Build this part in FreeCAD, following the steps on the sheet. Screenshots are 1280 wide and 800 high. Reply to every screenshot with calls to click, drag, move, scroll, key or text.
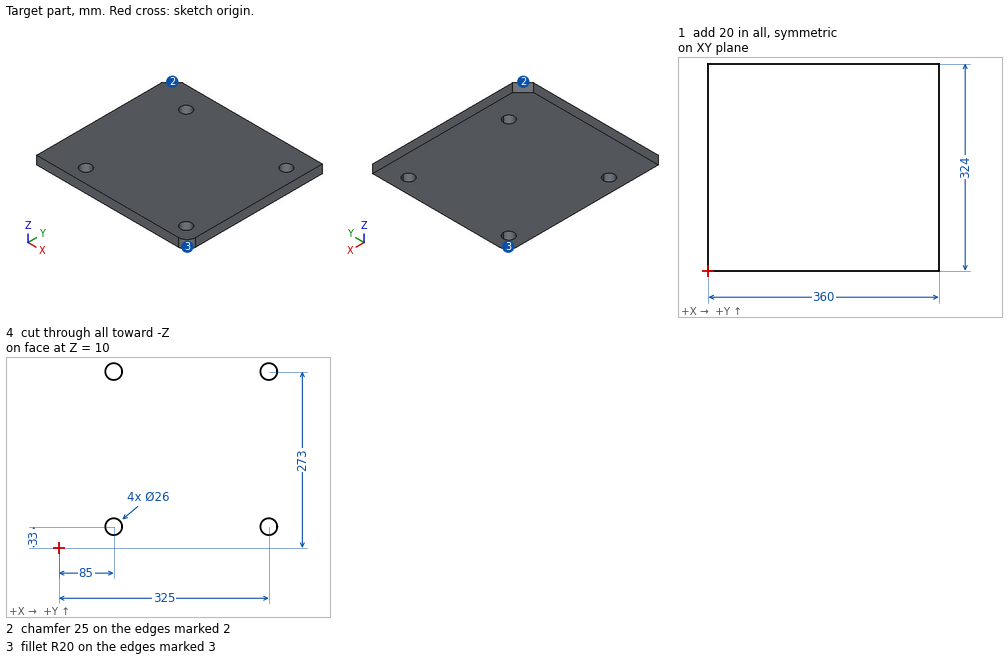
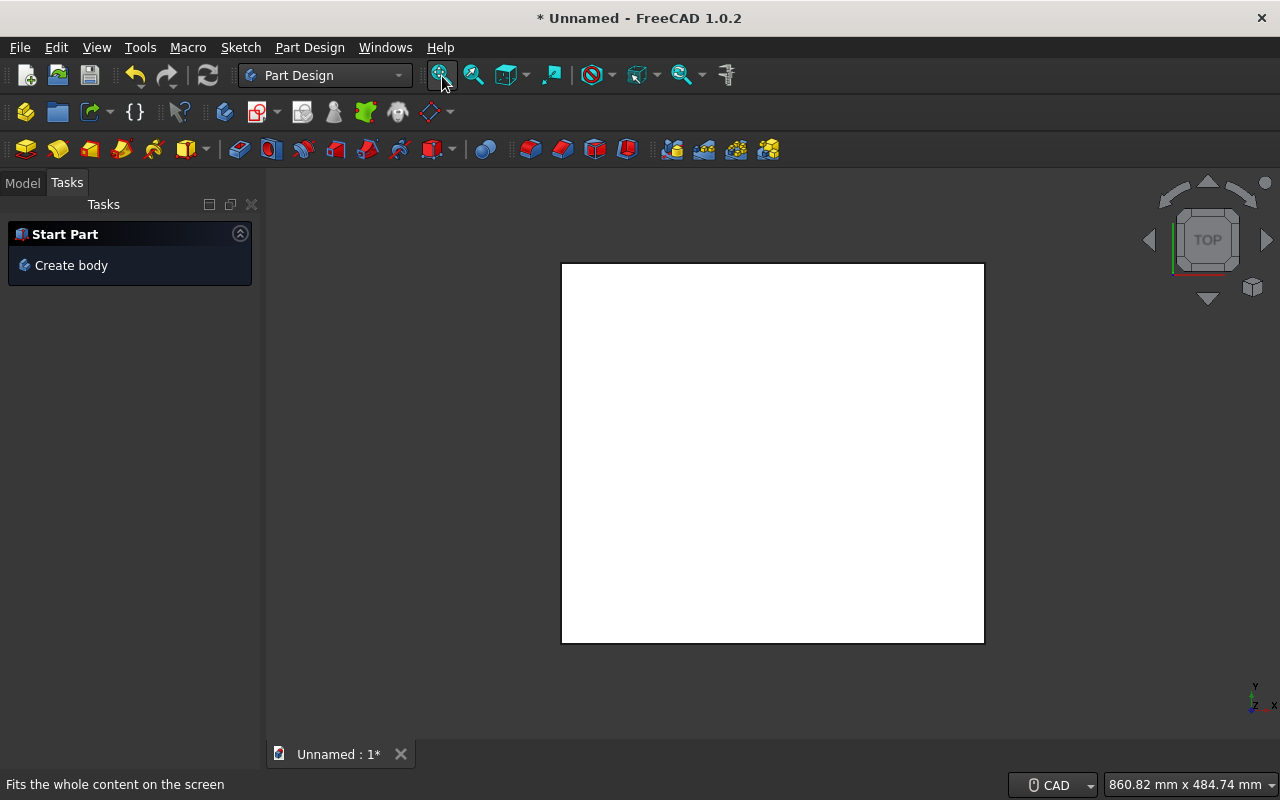
key(1)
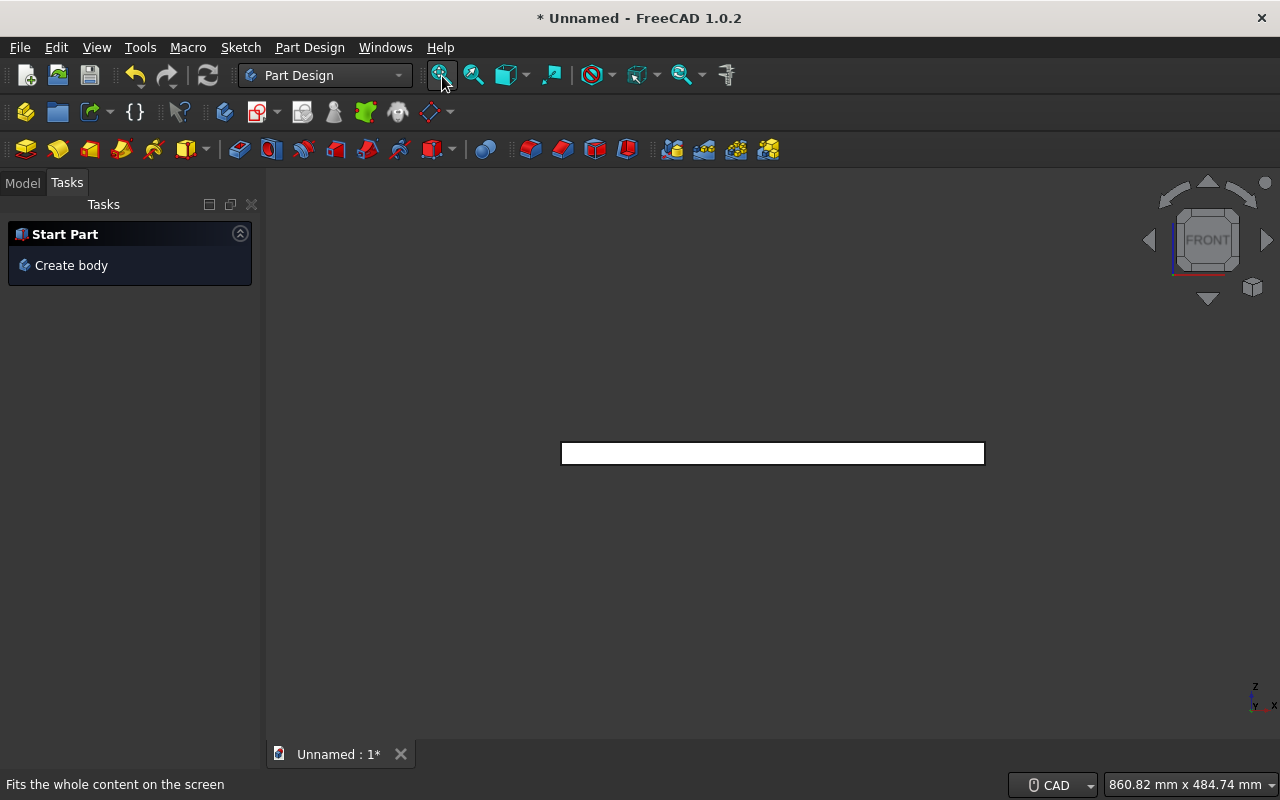
click(442, 76)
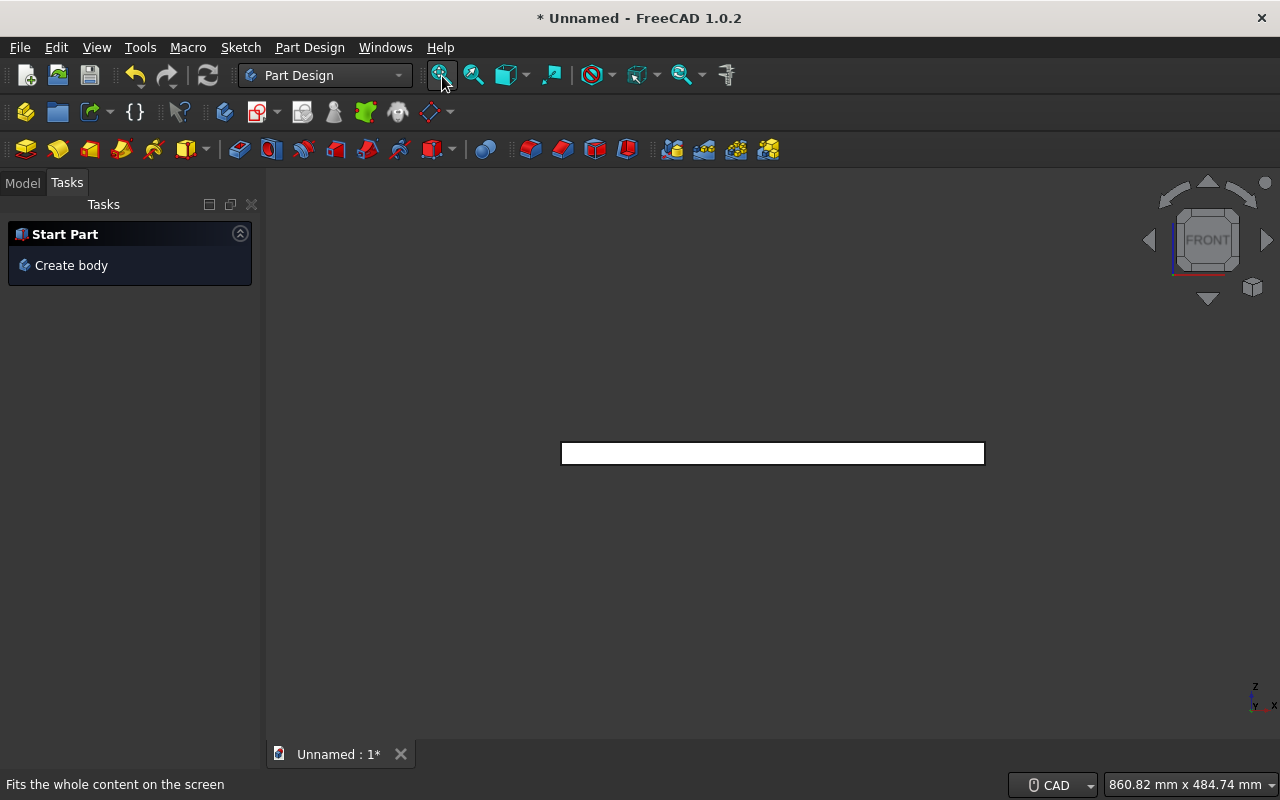
key(3)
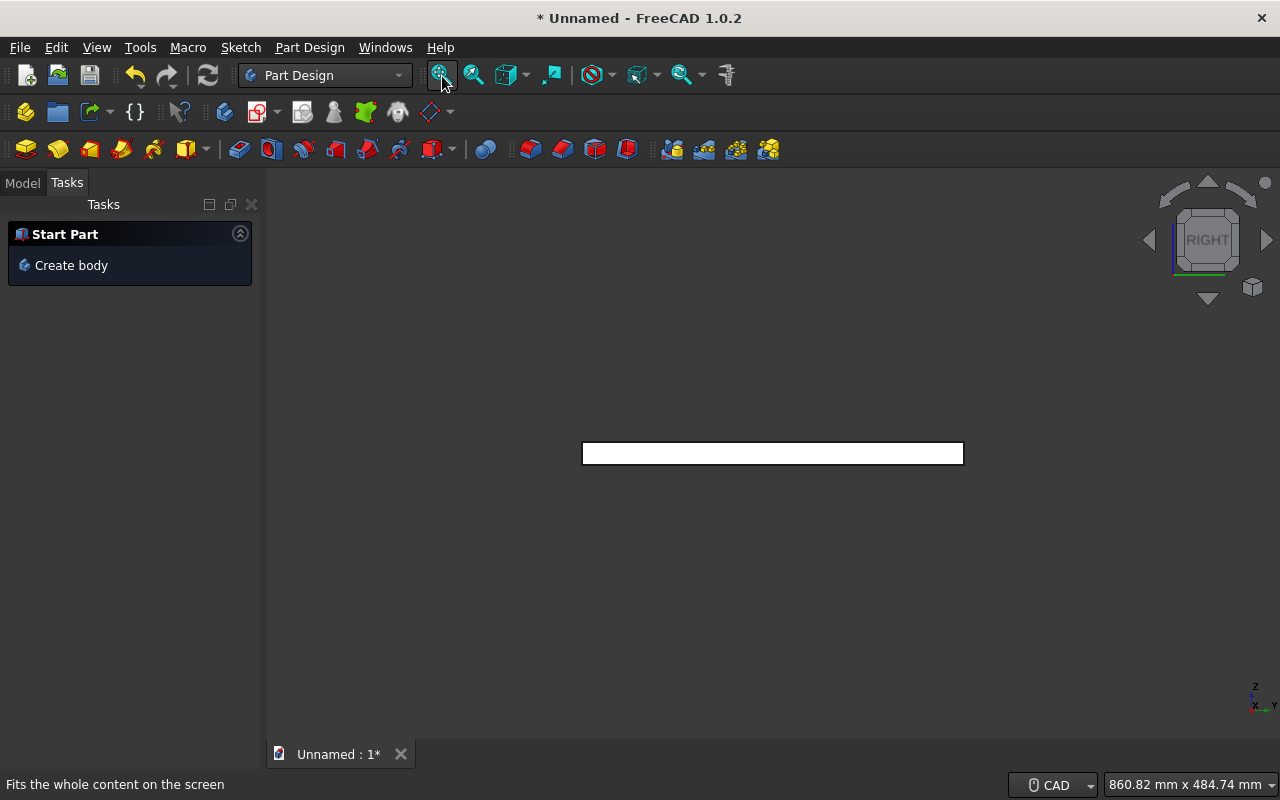
click(442, 76)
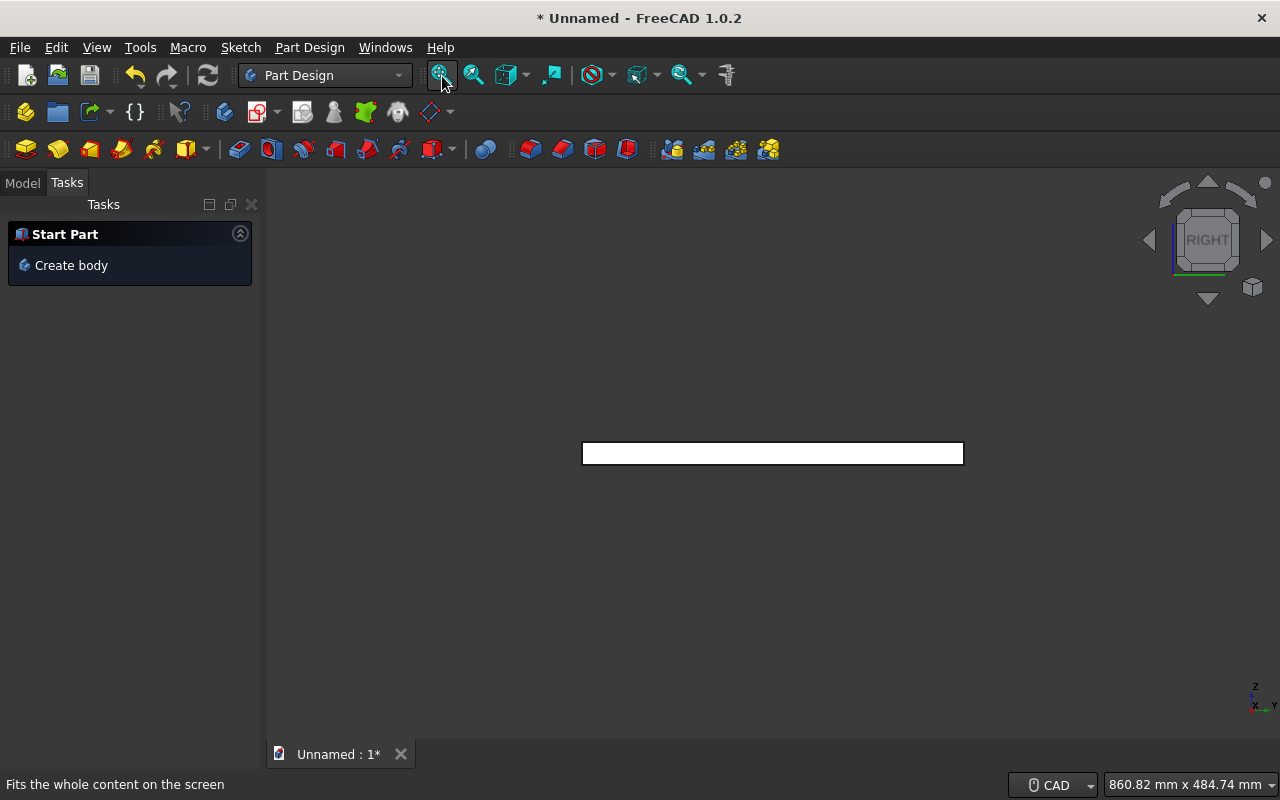
key(5)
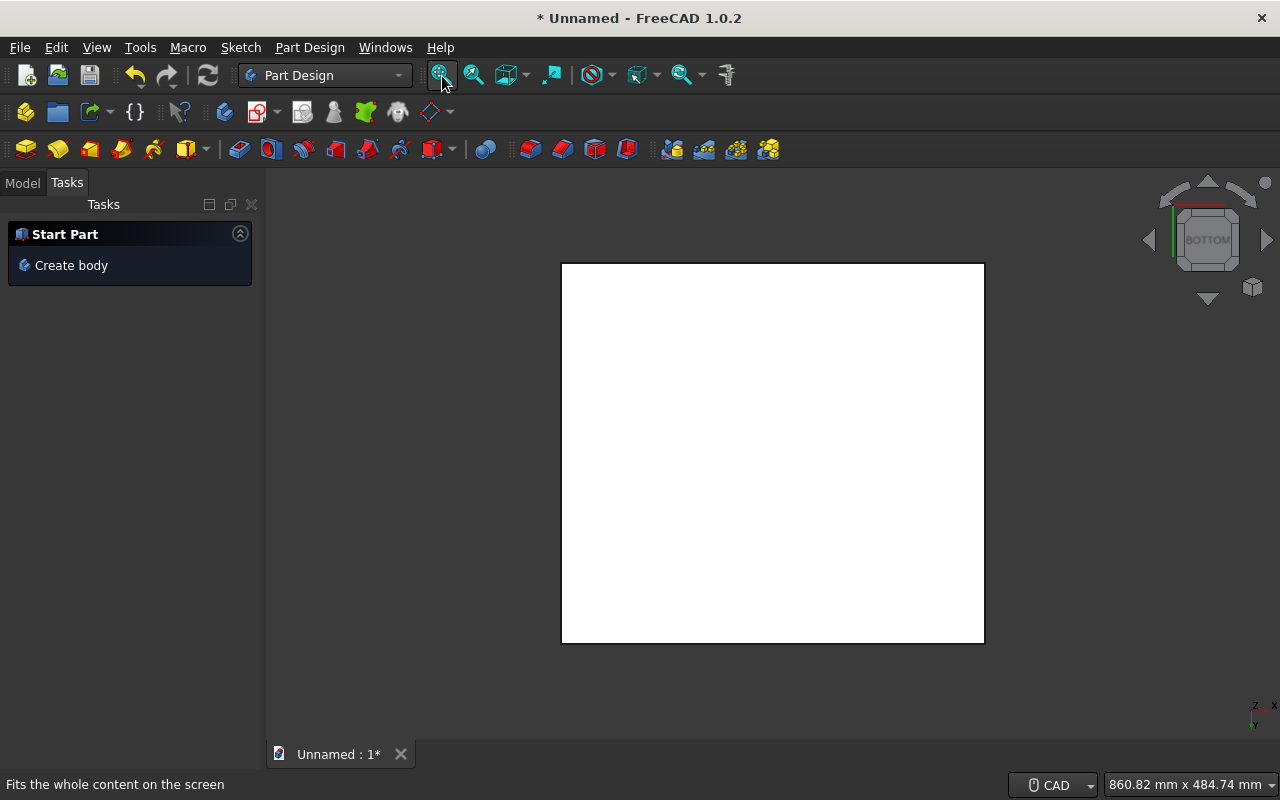
key(4)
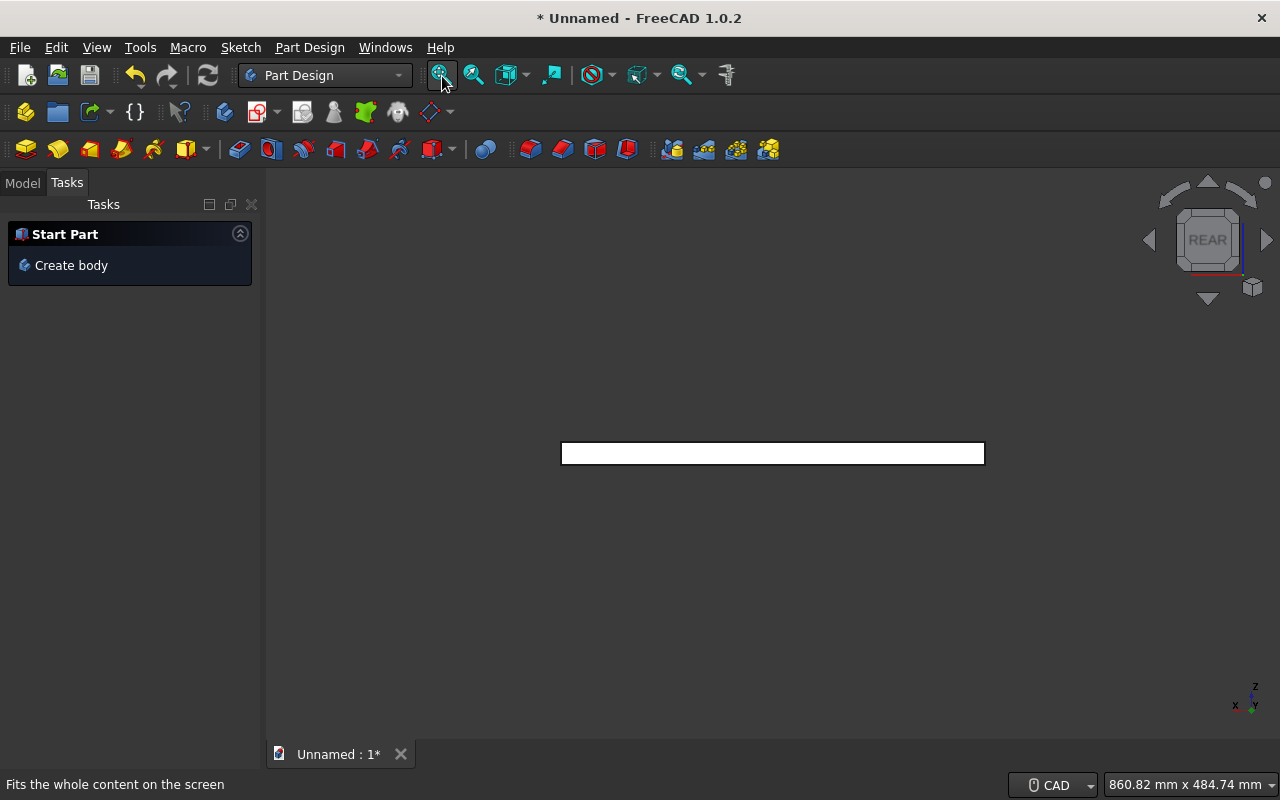
click(442, 76)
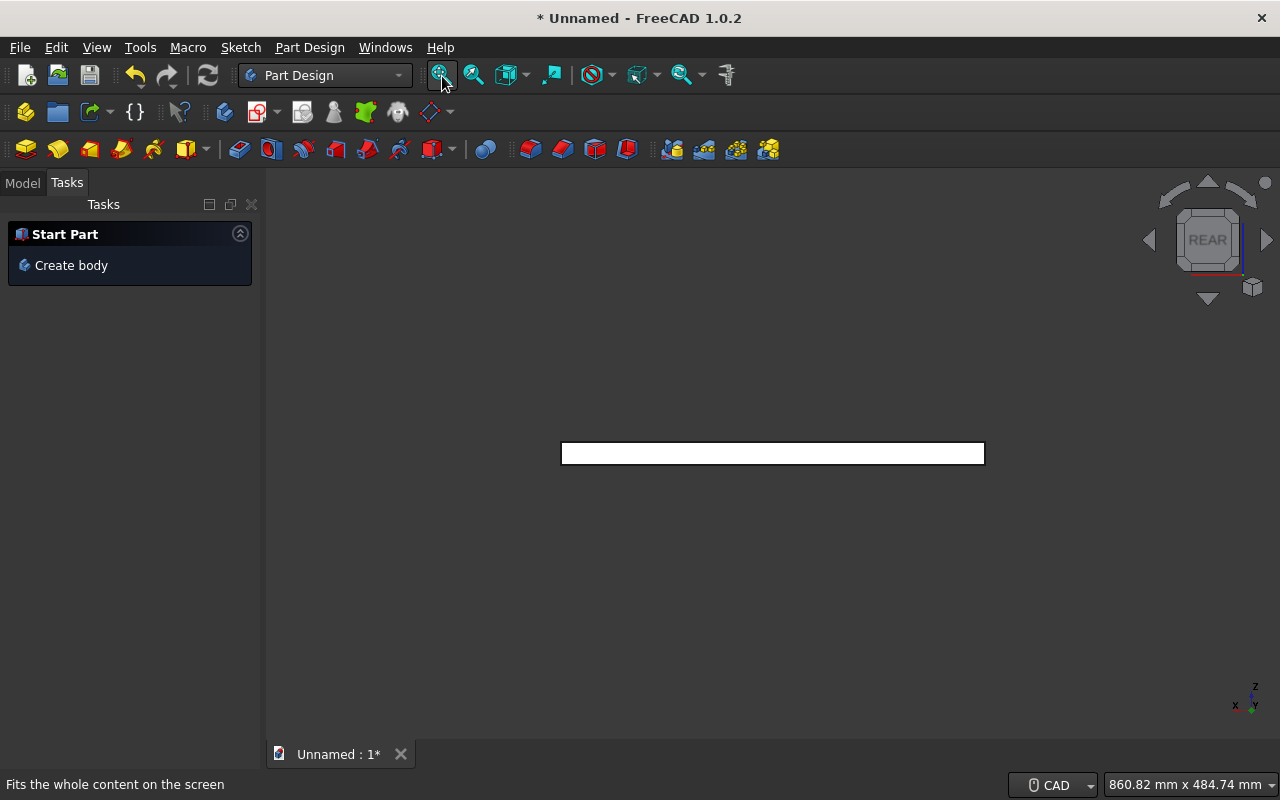
click(985, 453)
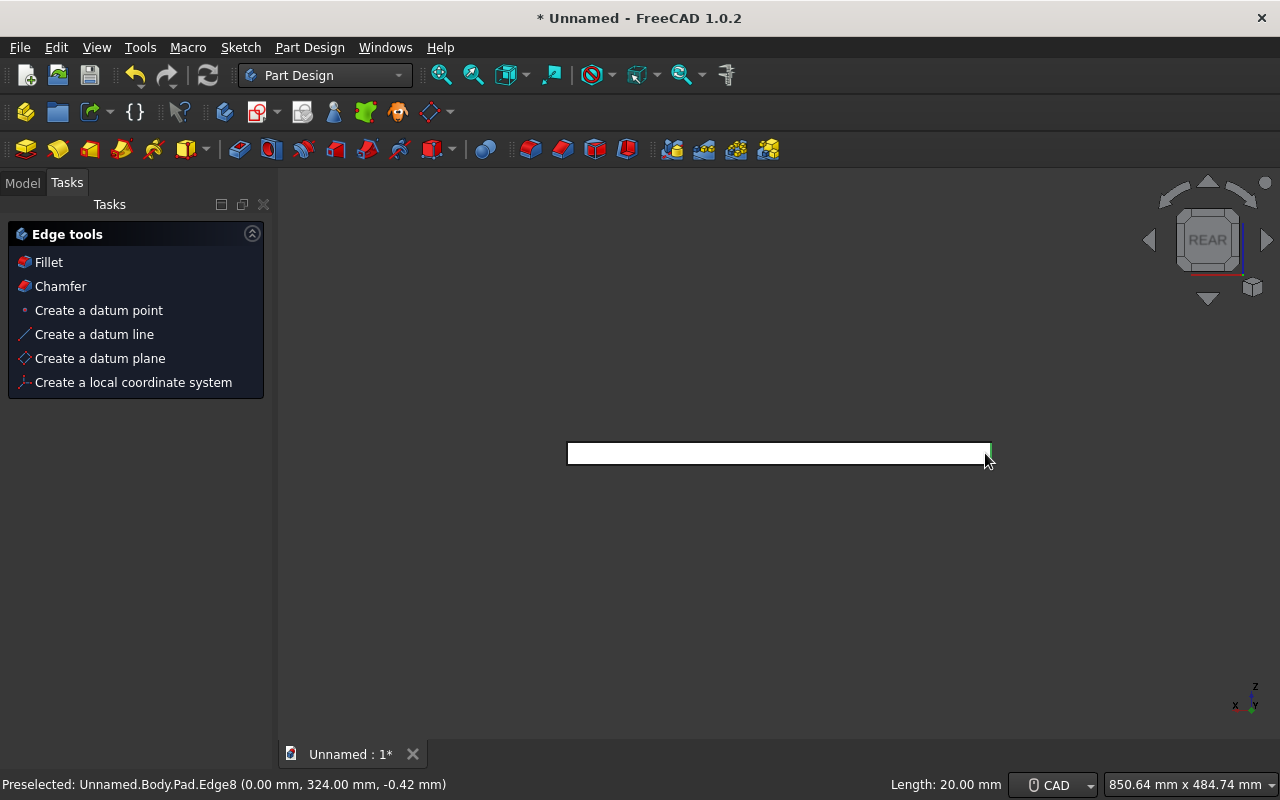
click(564, 150)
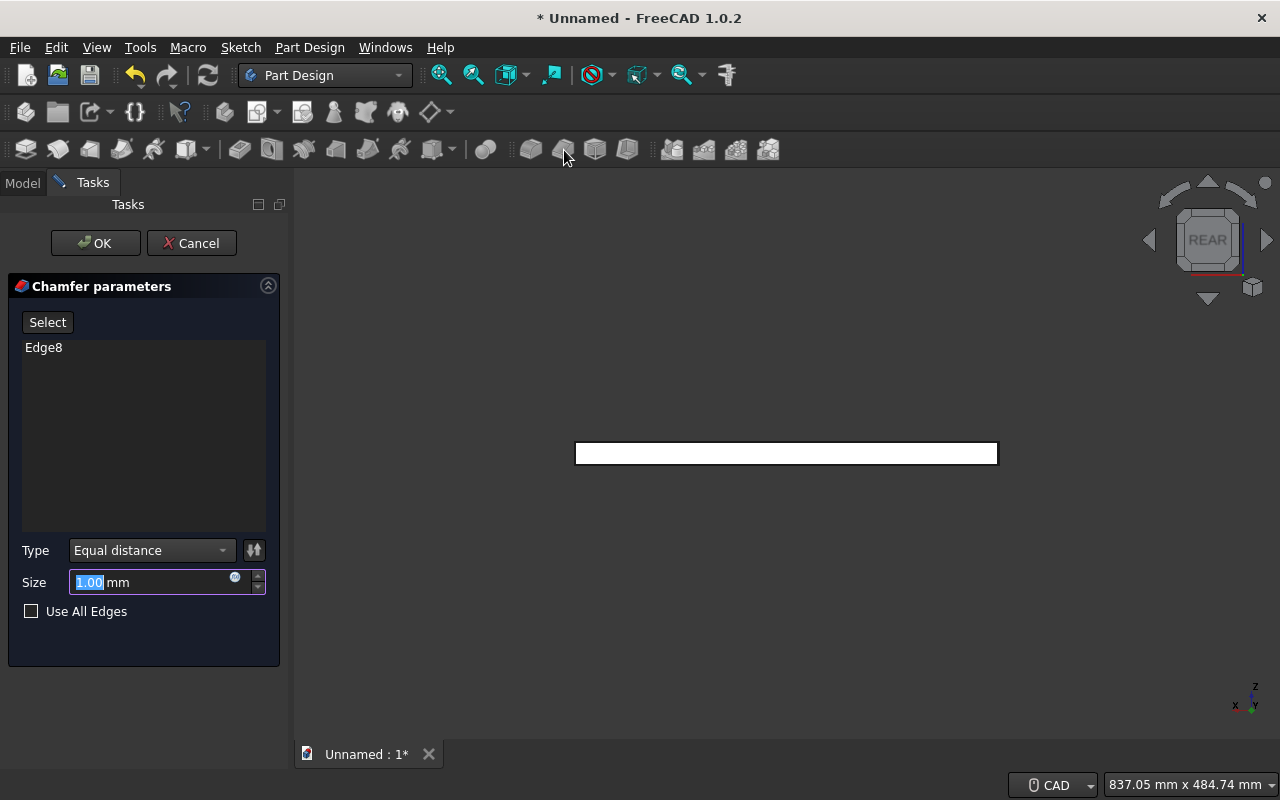
text(25)
key(Tab)